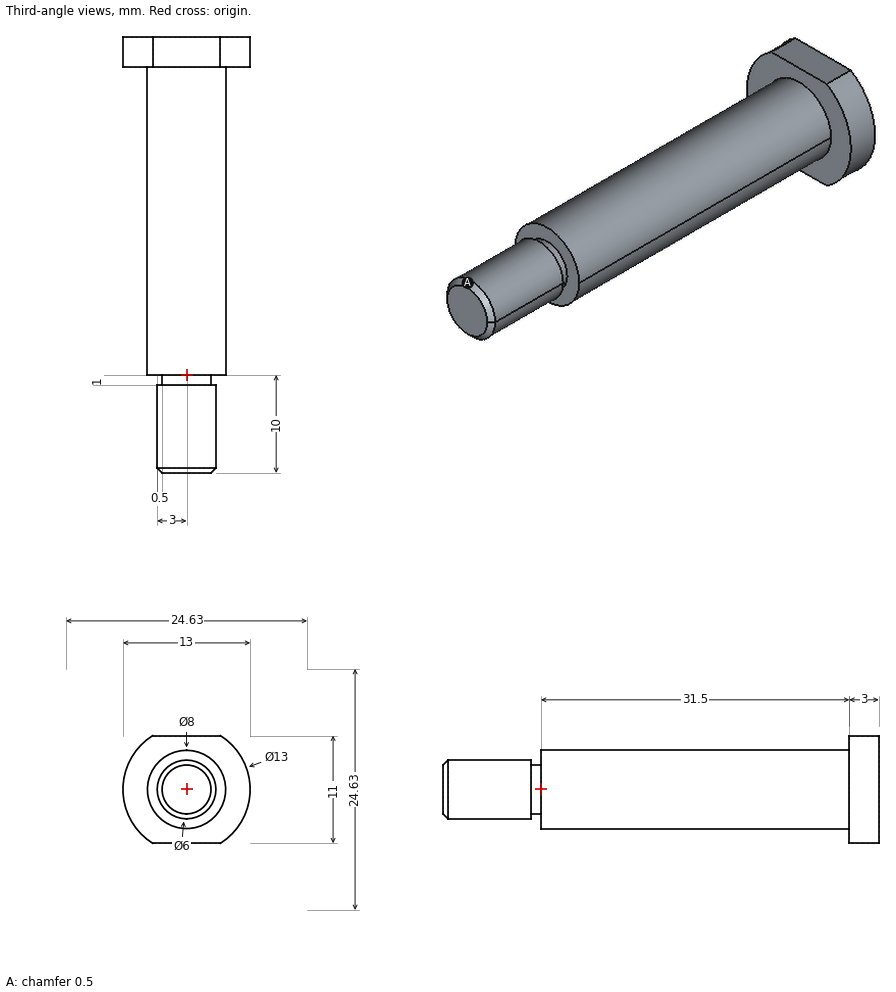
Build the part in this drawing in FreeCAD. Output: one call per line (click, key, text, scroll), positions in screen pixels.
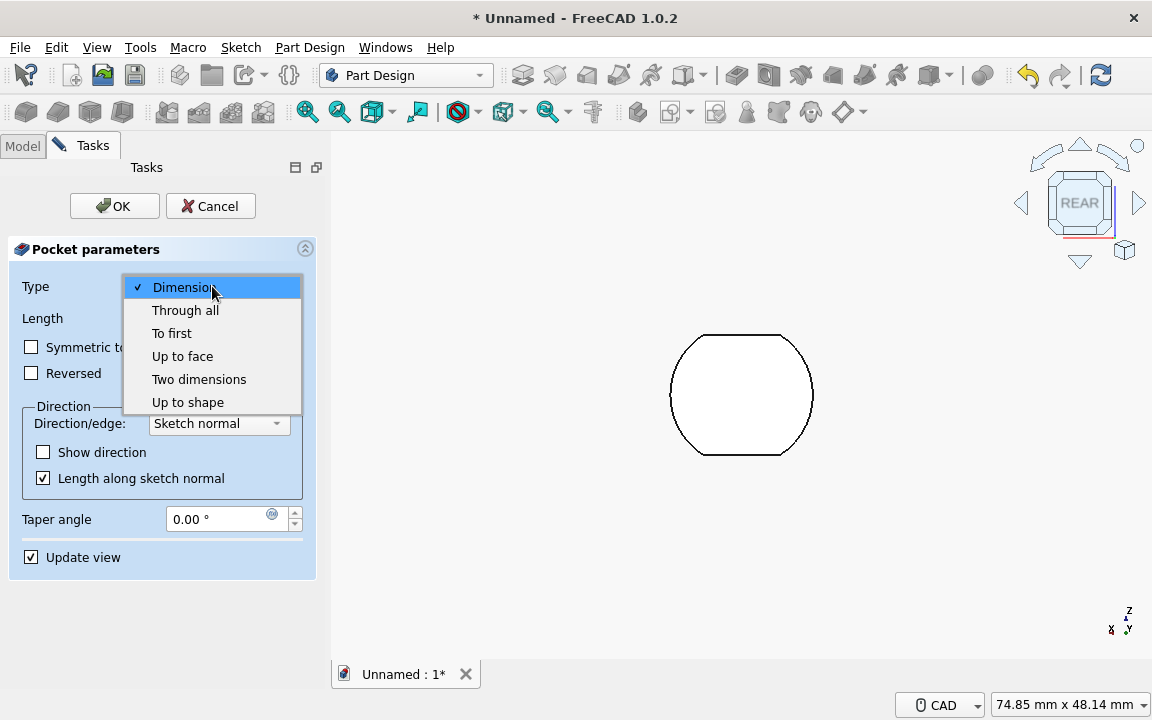
click(212, 310)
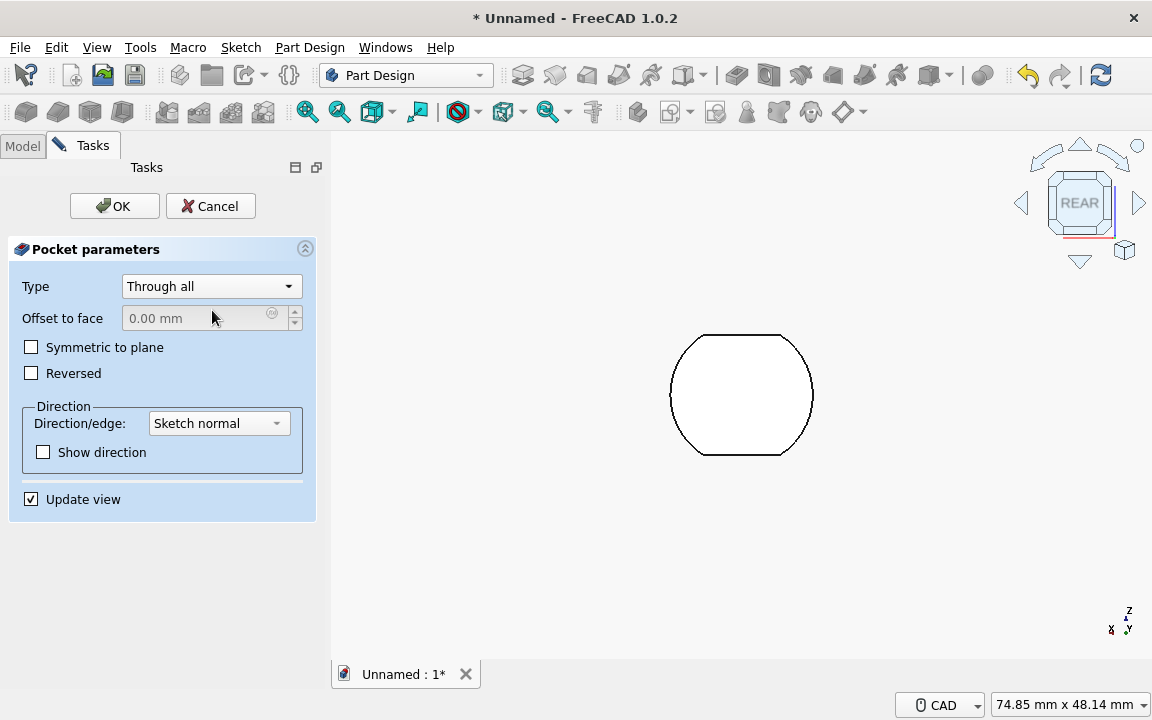
click(115, 206)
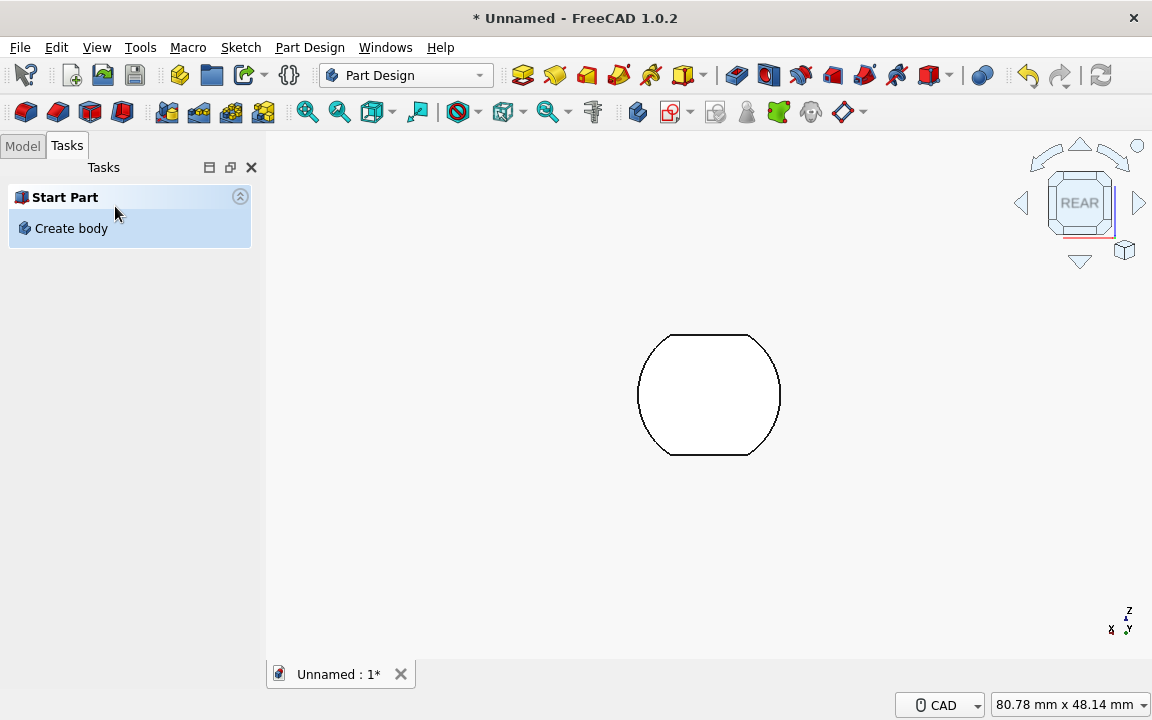
key(v)
key(f)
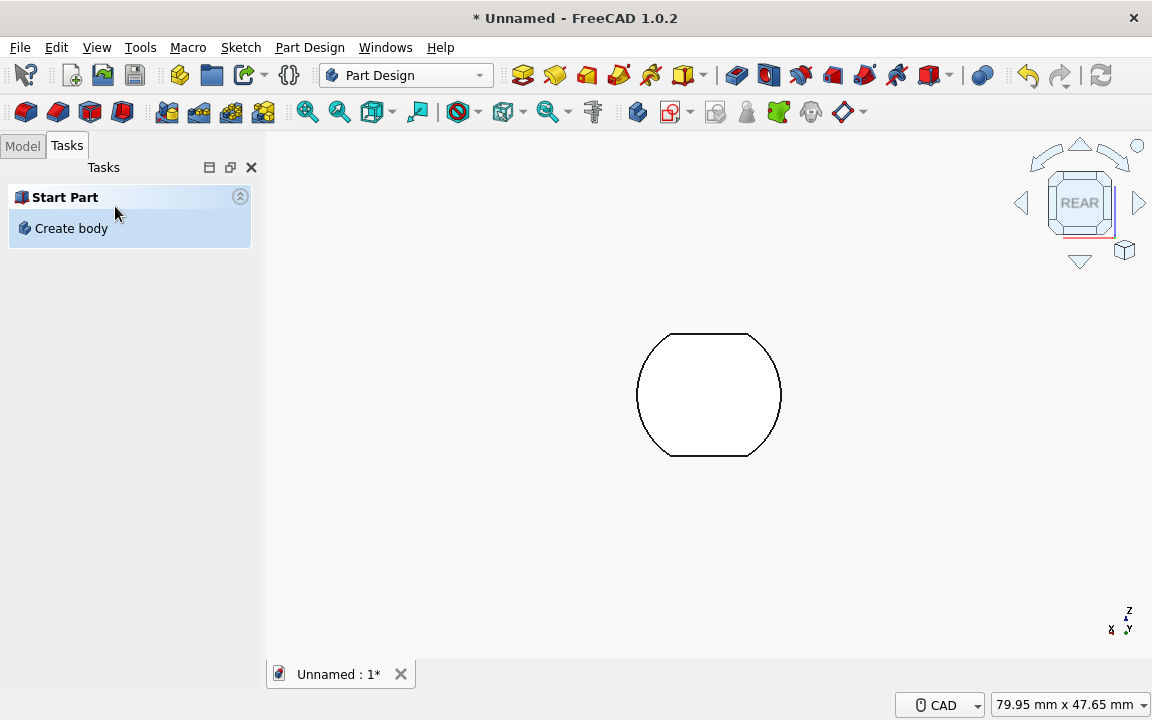
key(0)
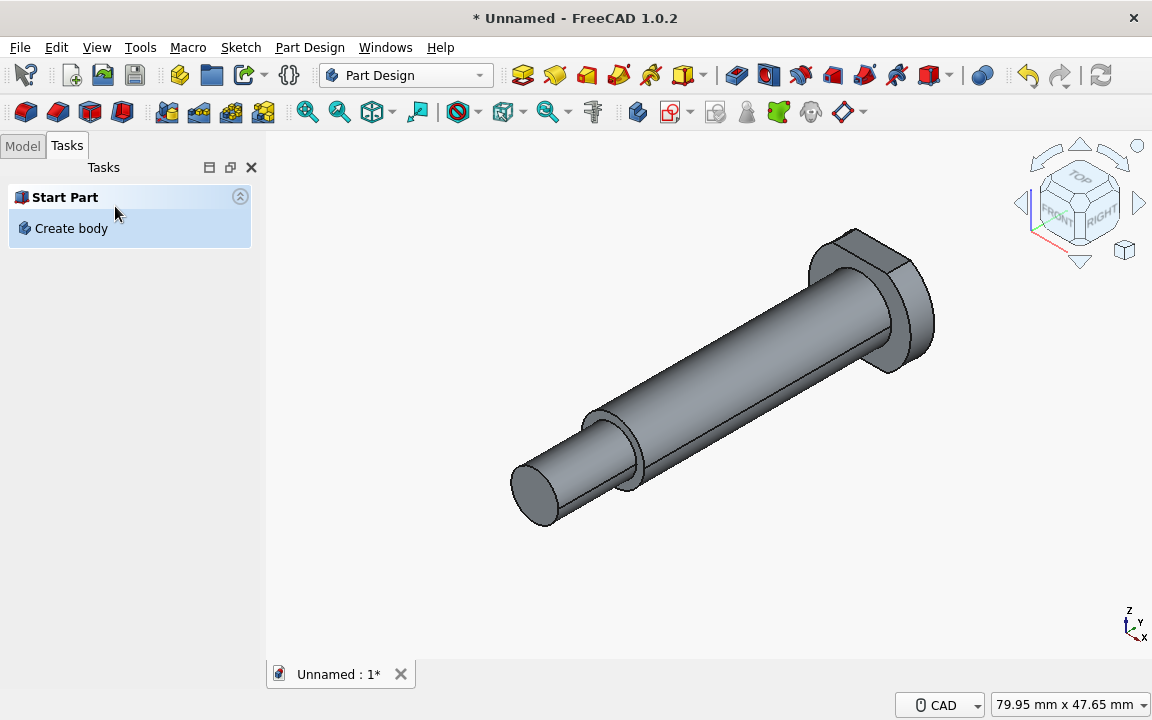
click(527, 465)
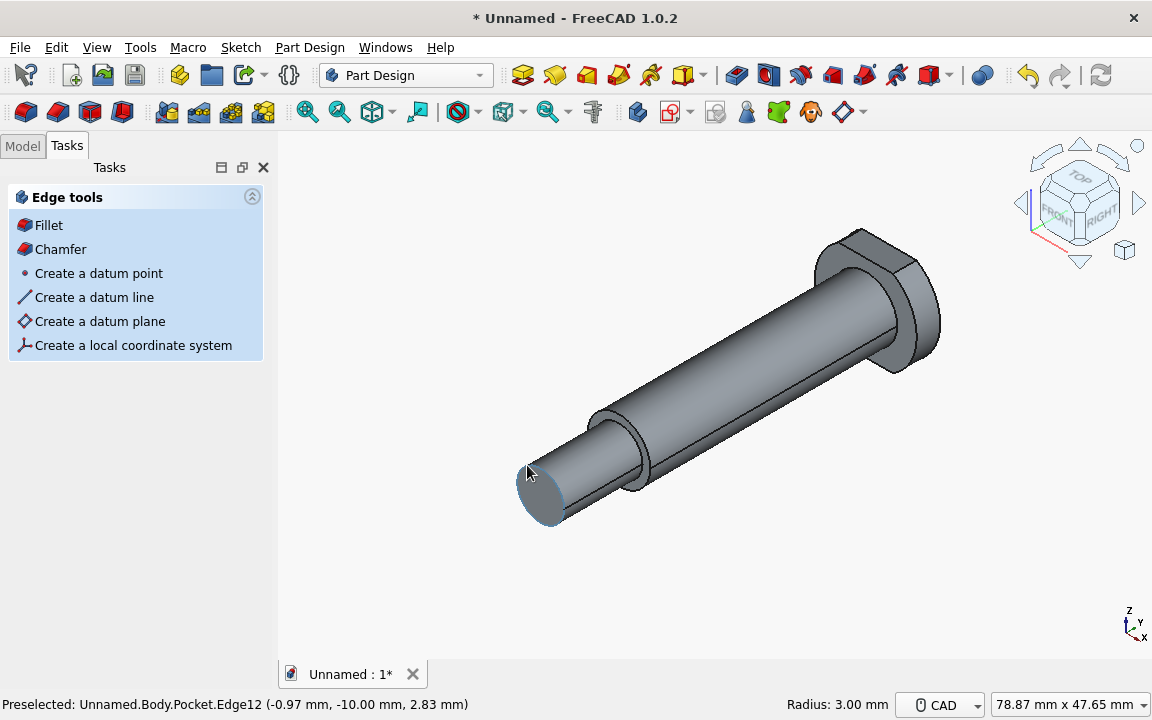
click(58, 112)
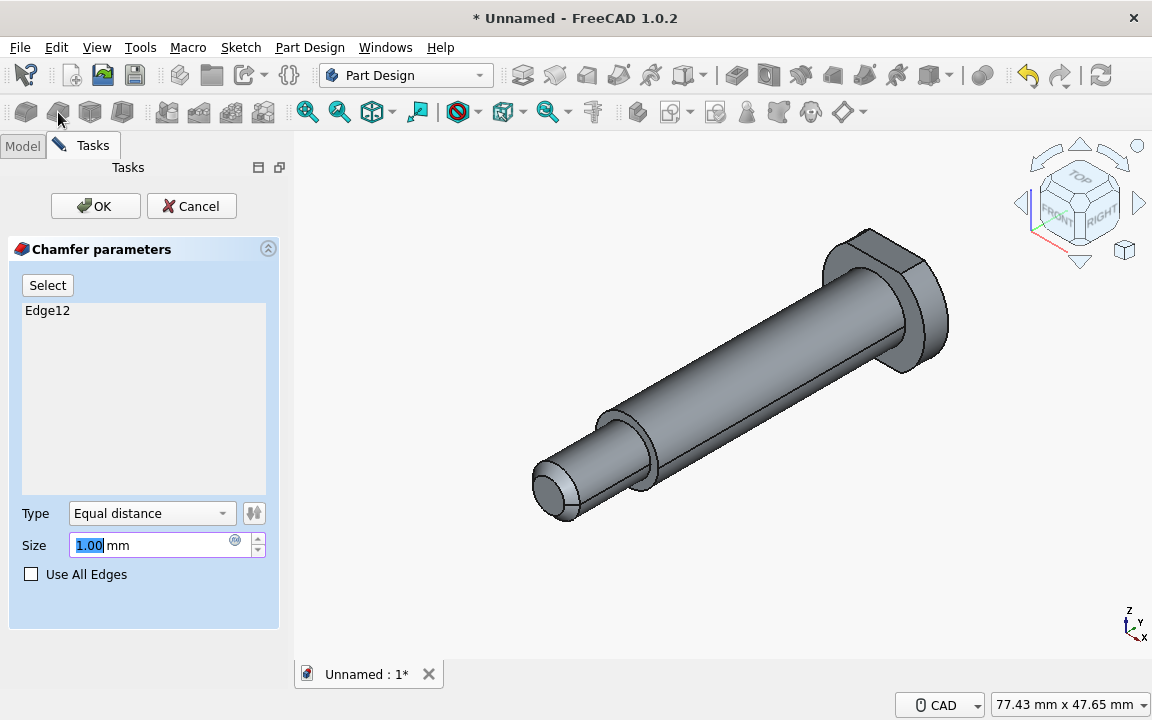
text(0.5)
key(Tab)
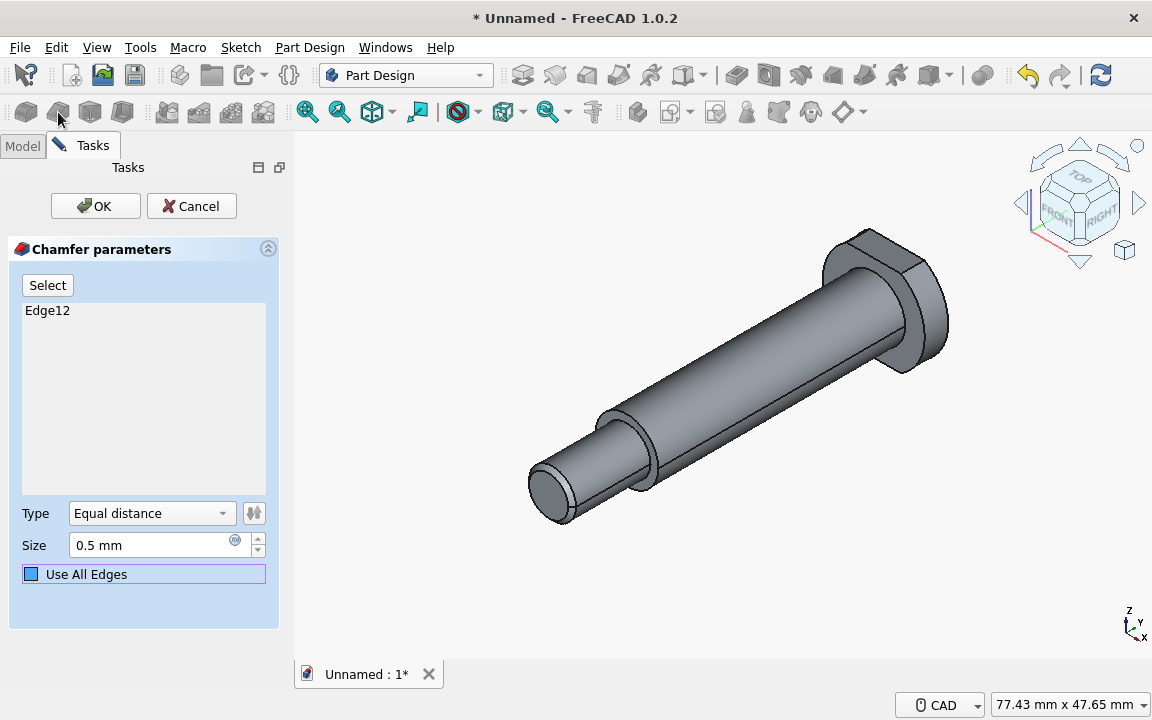
click(96, 206)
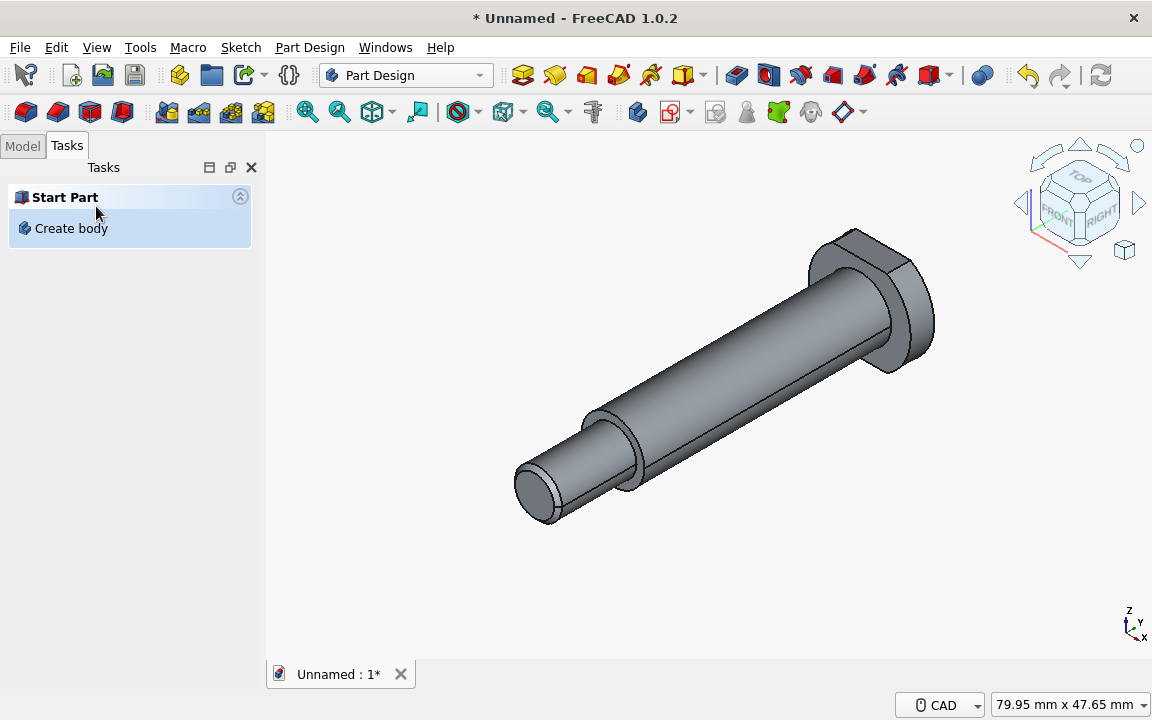
click(670, 112)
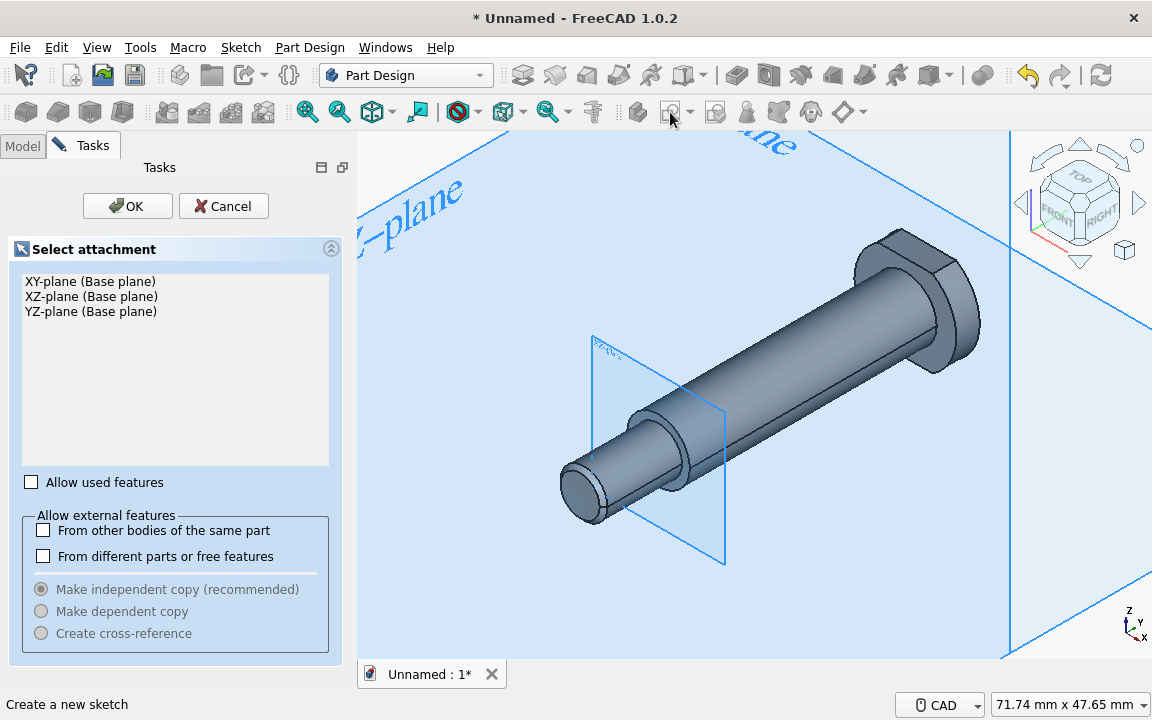
click(82, 282)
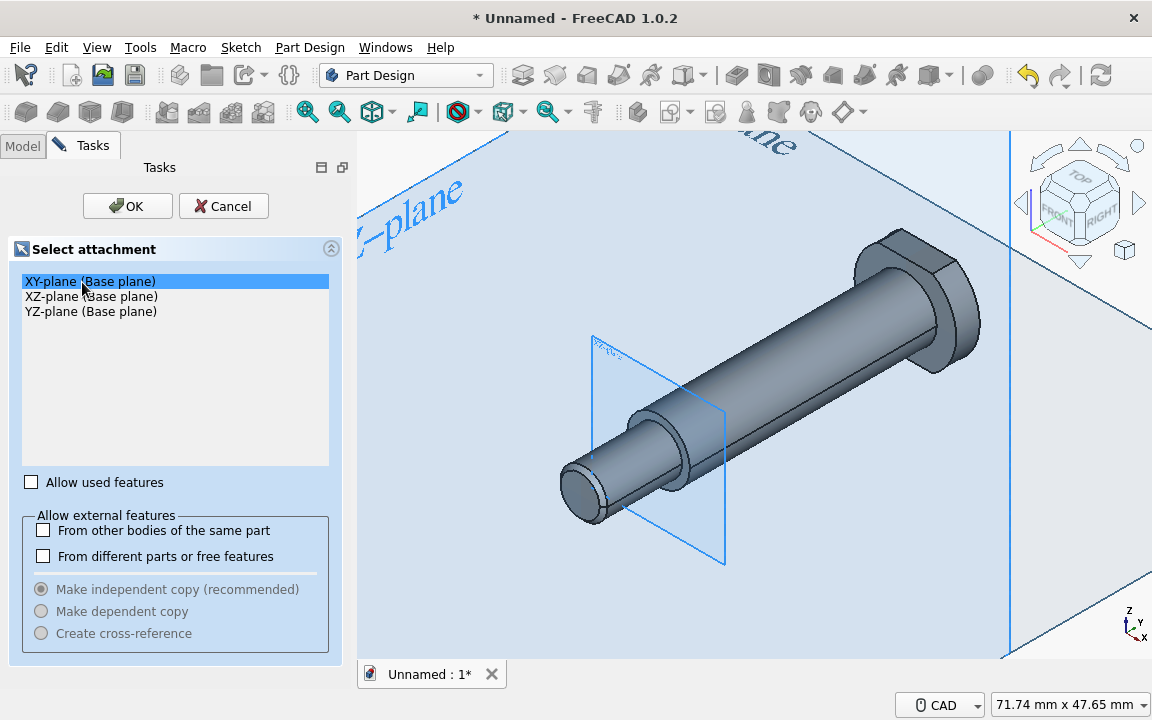
click(128, 206)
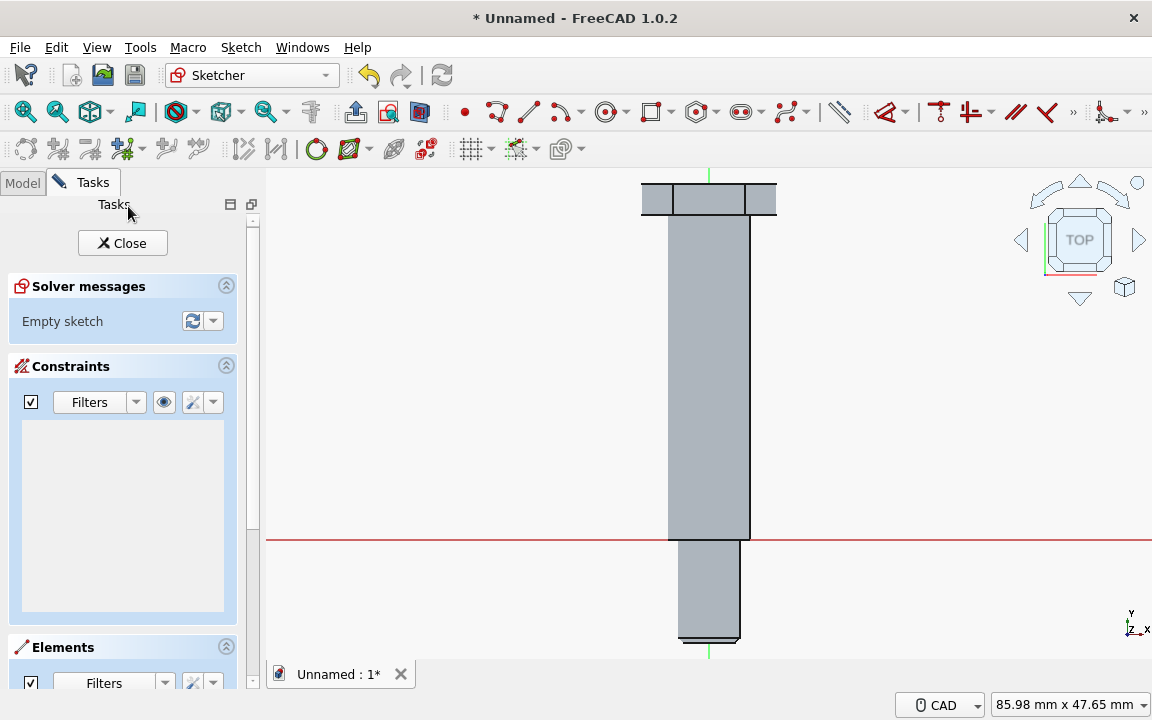
key(q)
key(s)